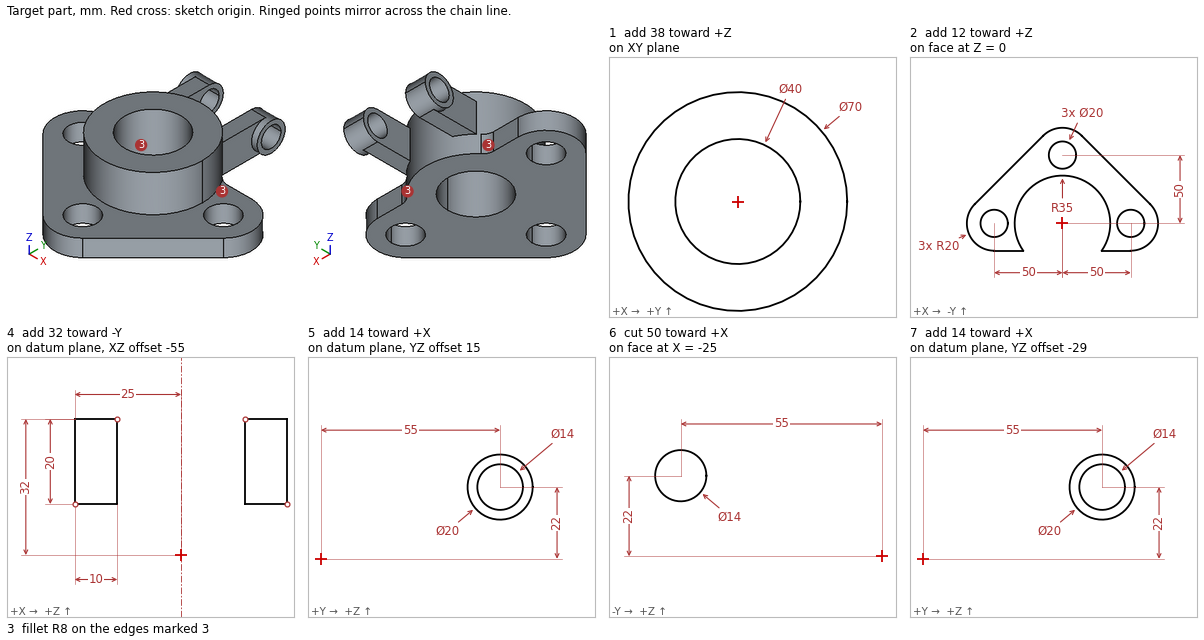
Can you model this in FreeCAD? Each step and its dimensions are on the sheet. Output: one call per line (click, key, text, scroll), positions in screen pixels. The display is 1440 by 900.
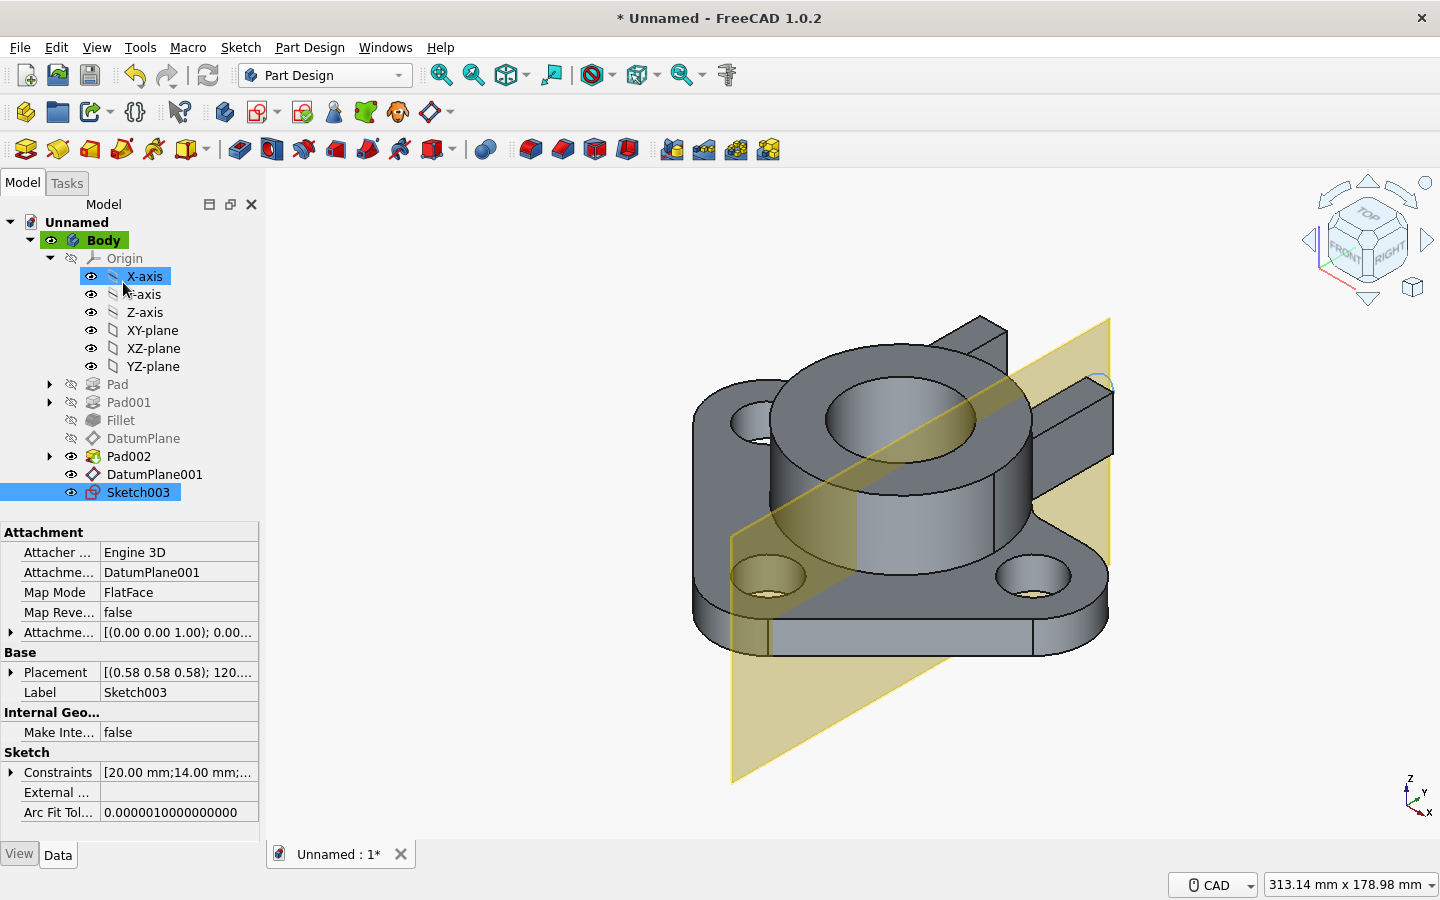
click(26, 150)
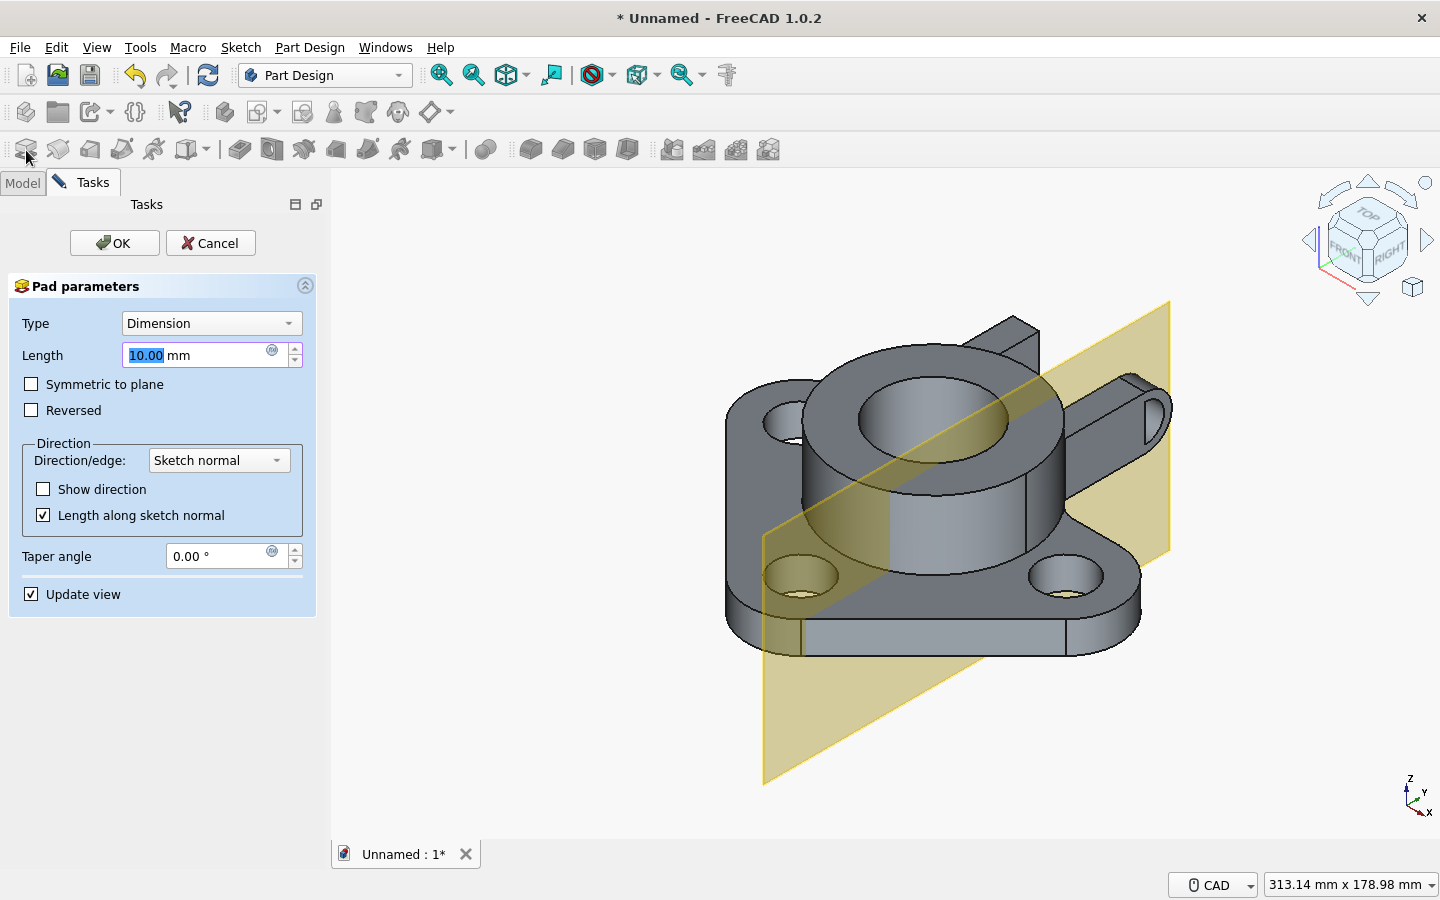
text(14)
key(Tab)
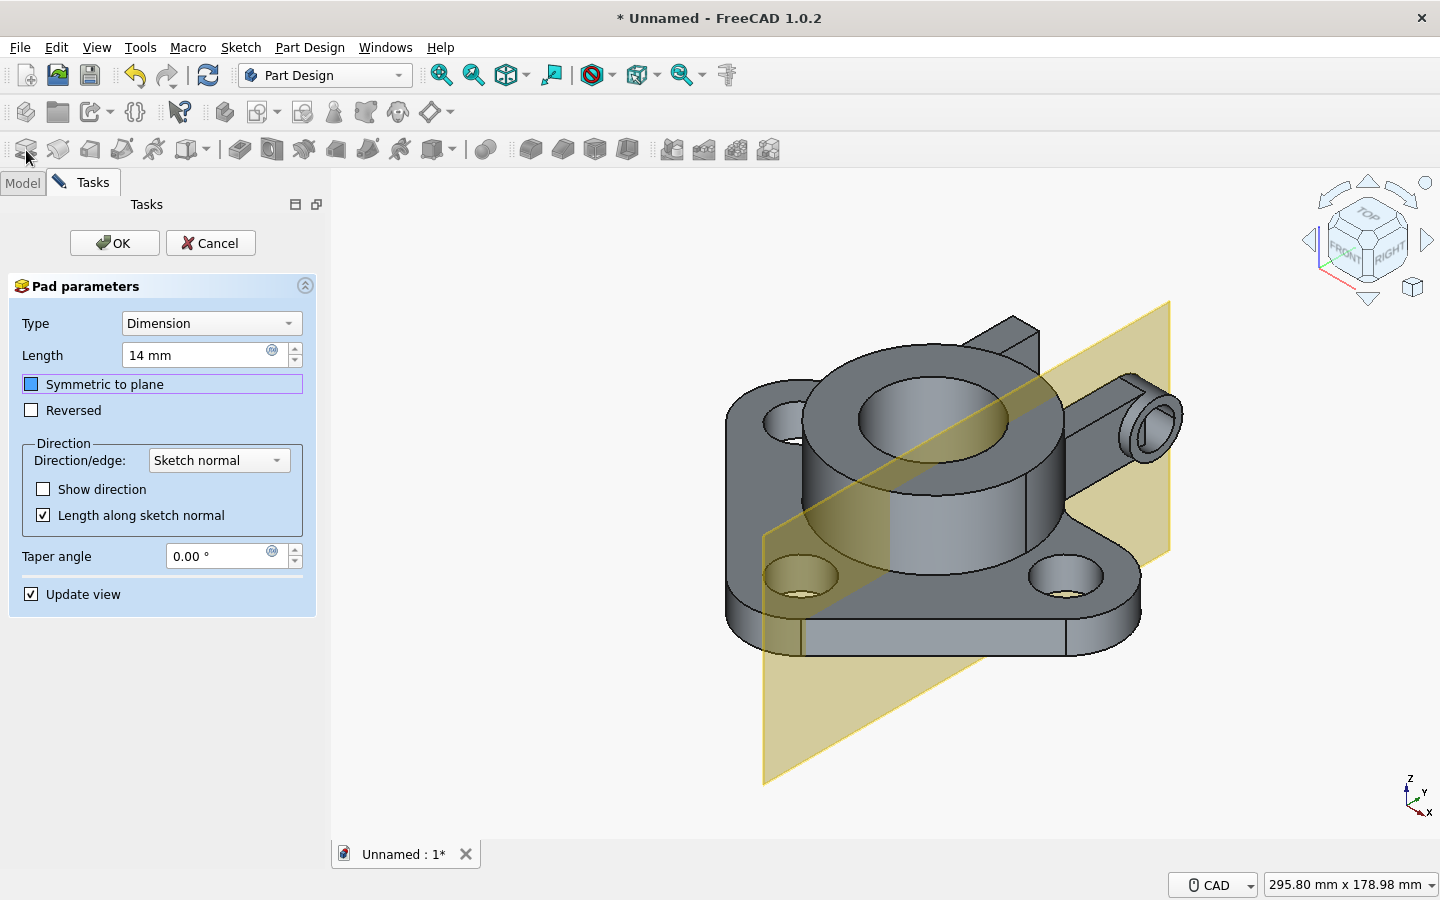
click(115, 243)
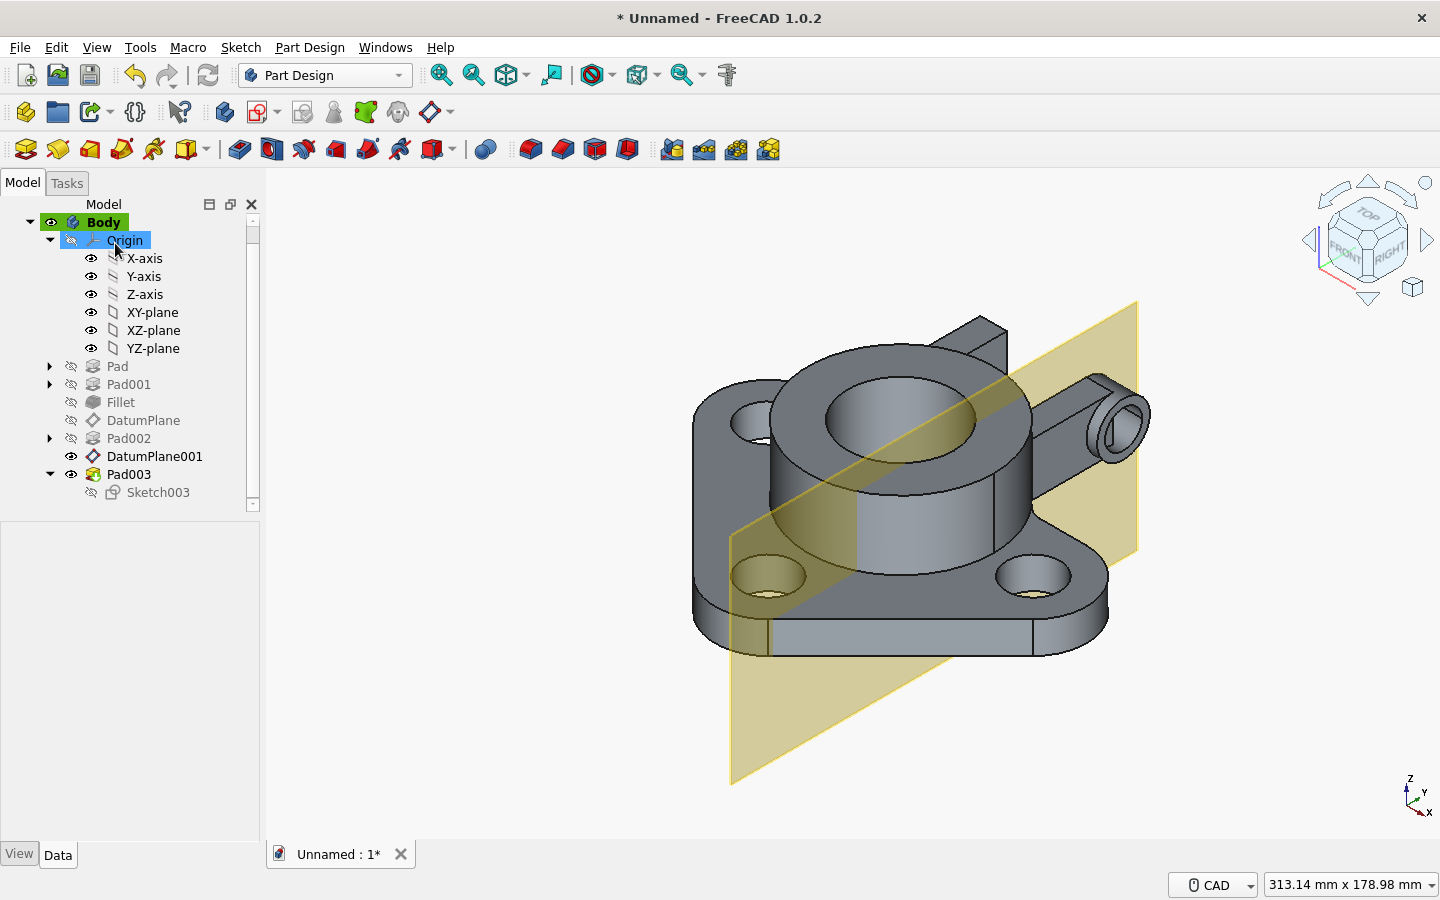
click(116, 456)
key(space)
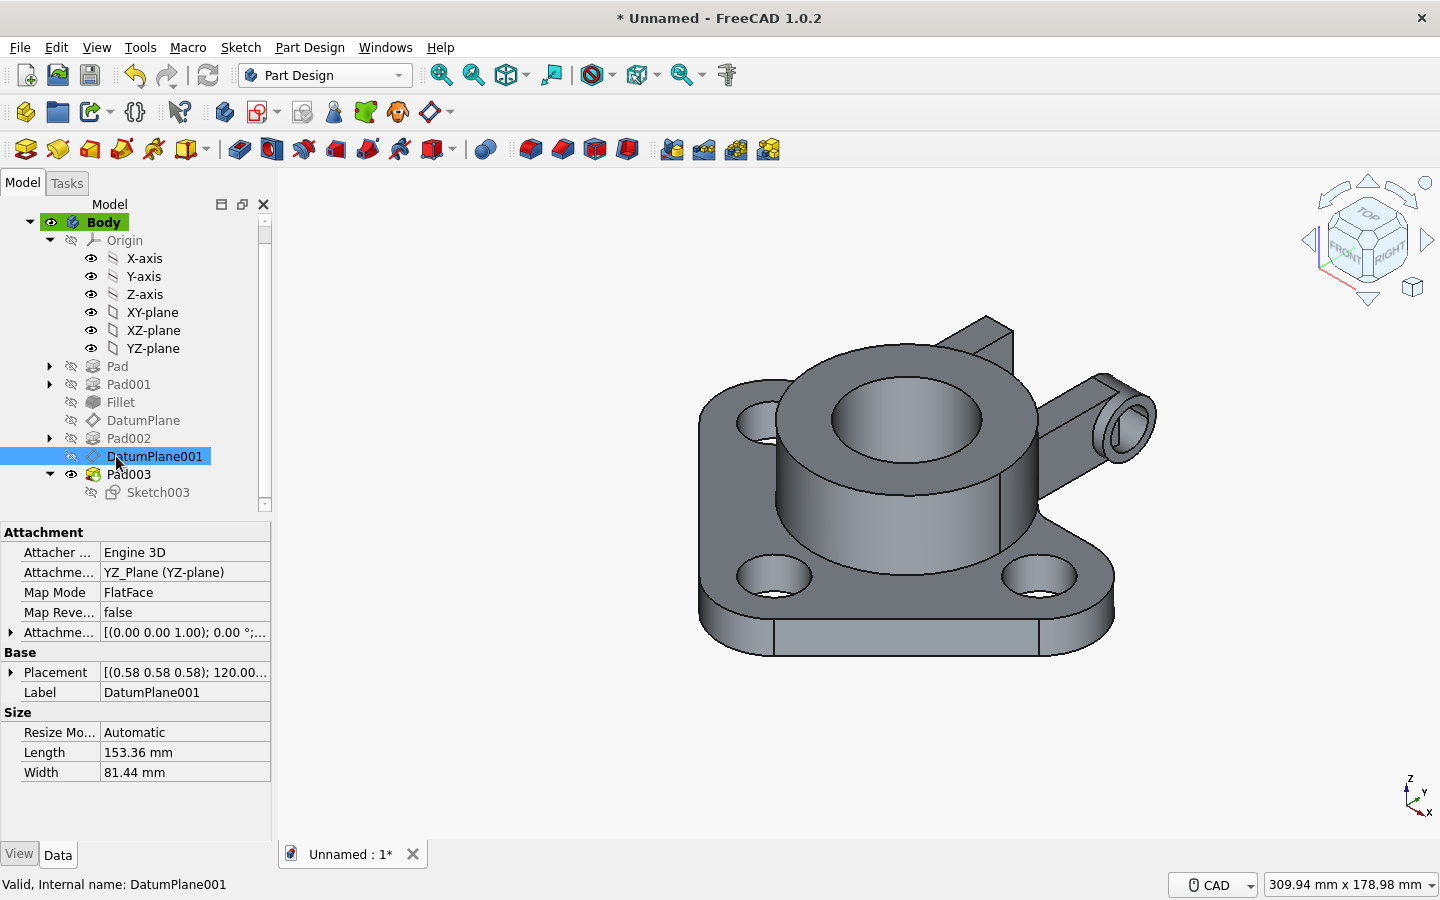
key(6)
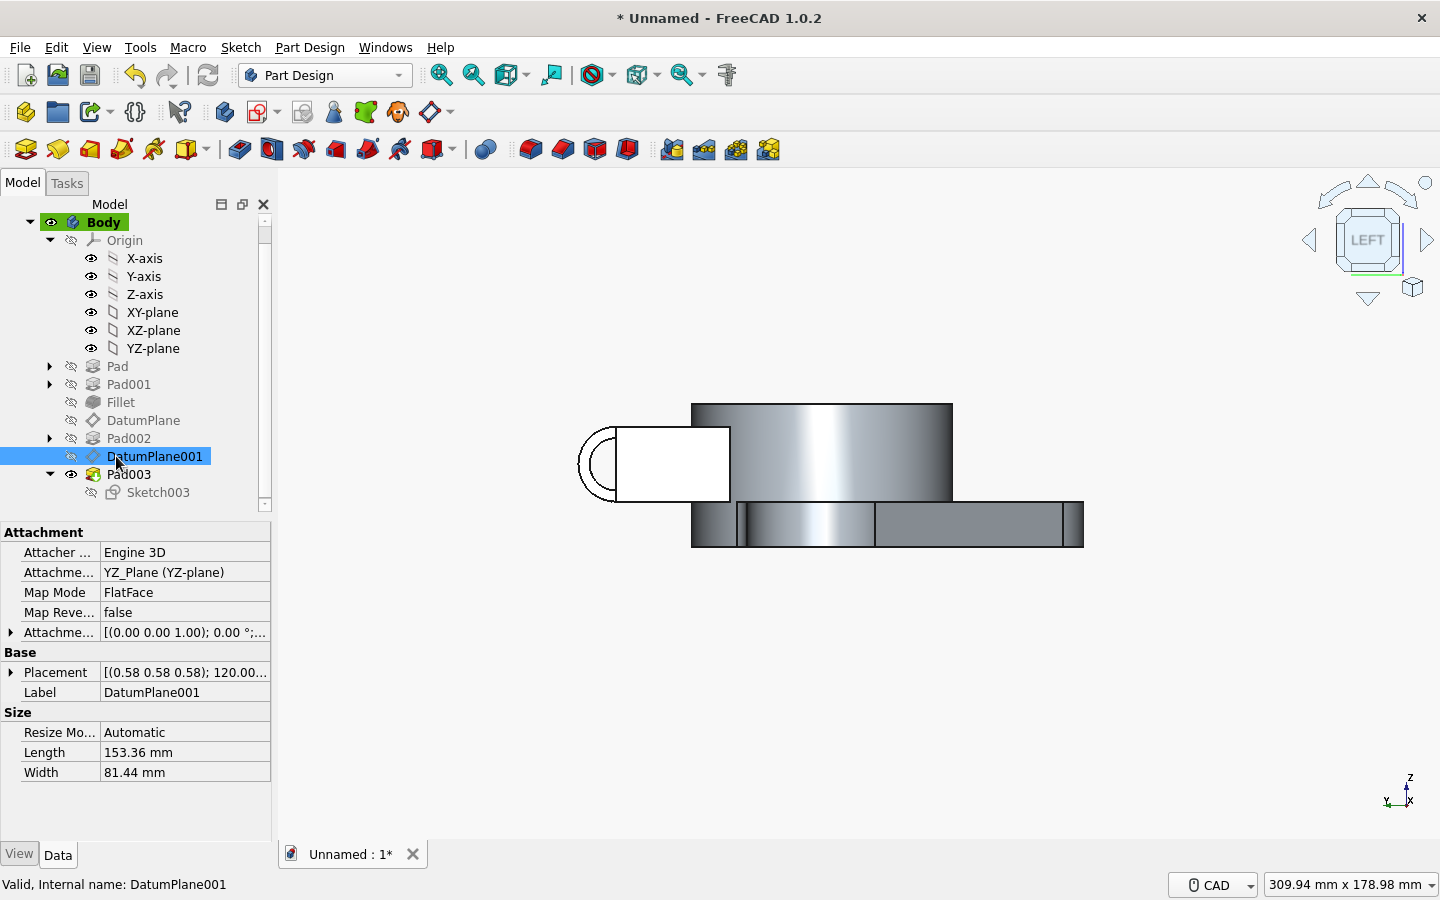
key(v)
key(f)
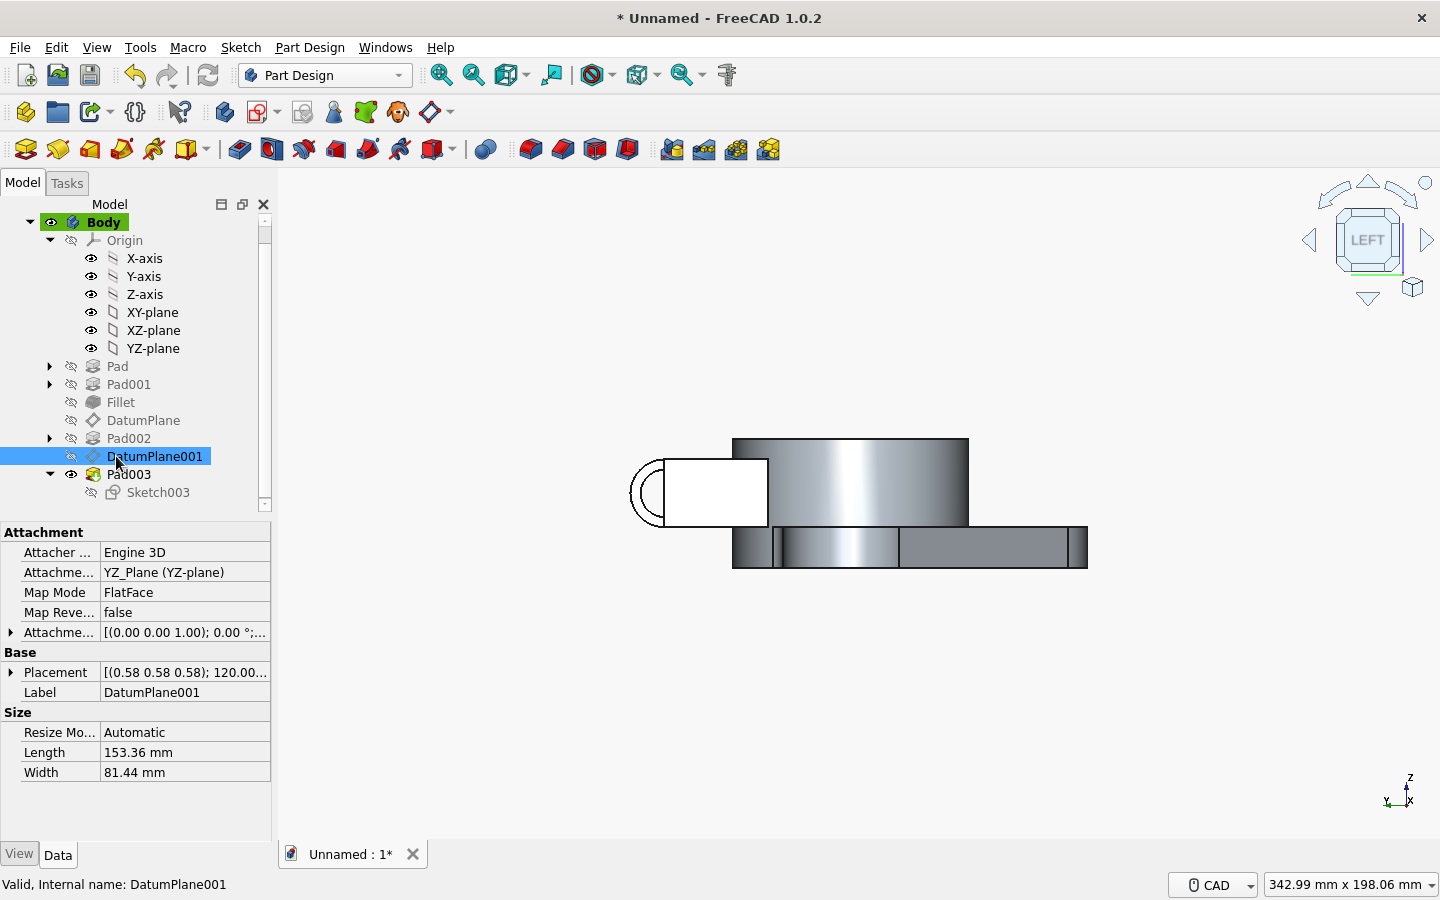
click(701, 492)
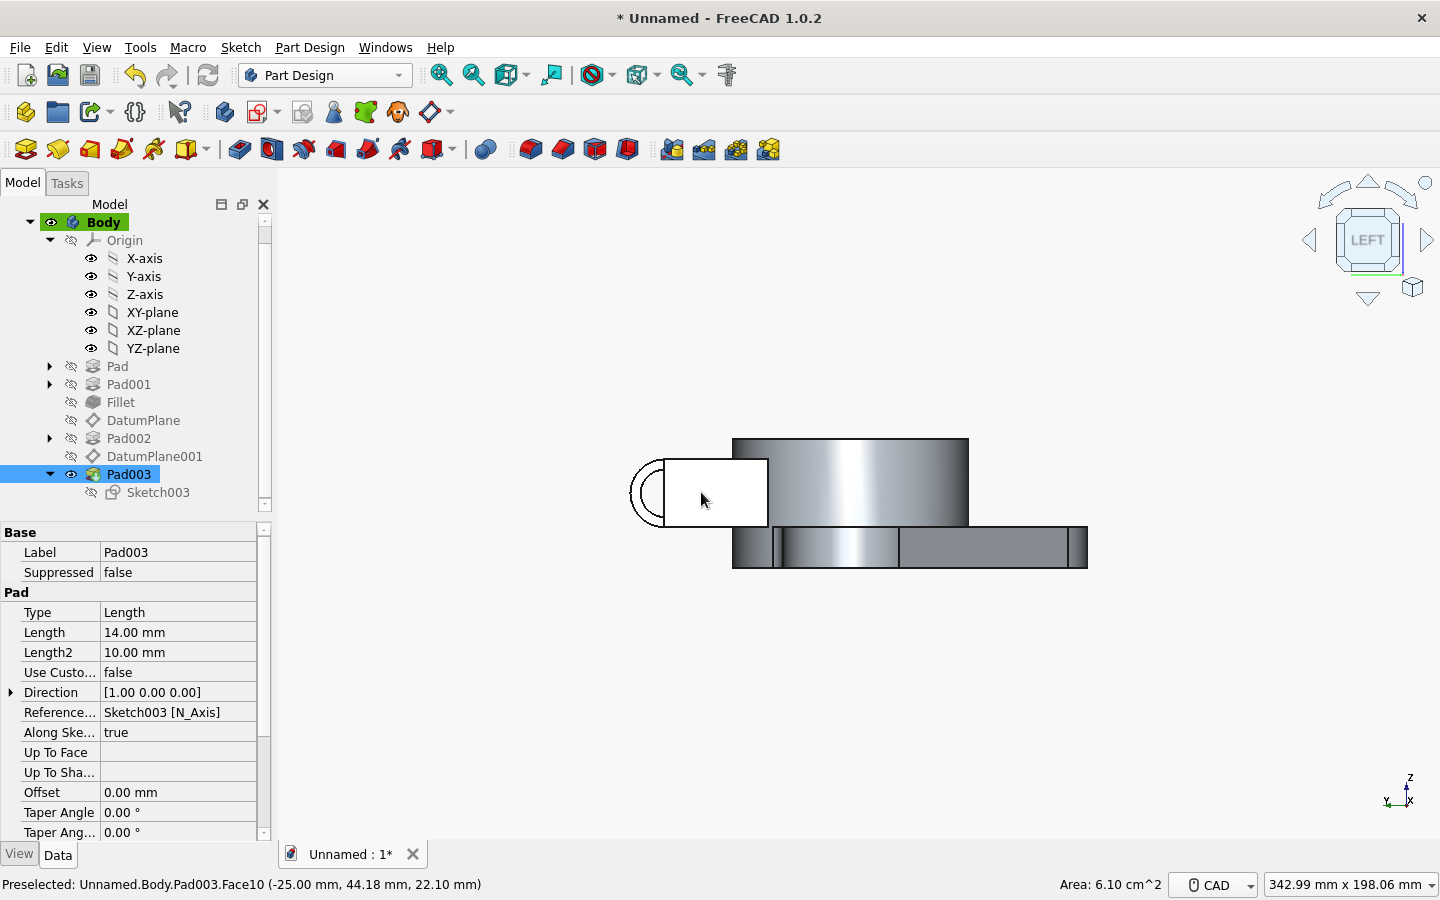
click(258, 112)